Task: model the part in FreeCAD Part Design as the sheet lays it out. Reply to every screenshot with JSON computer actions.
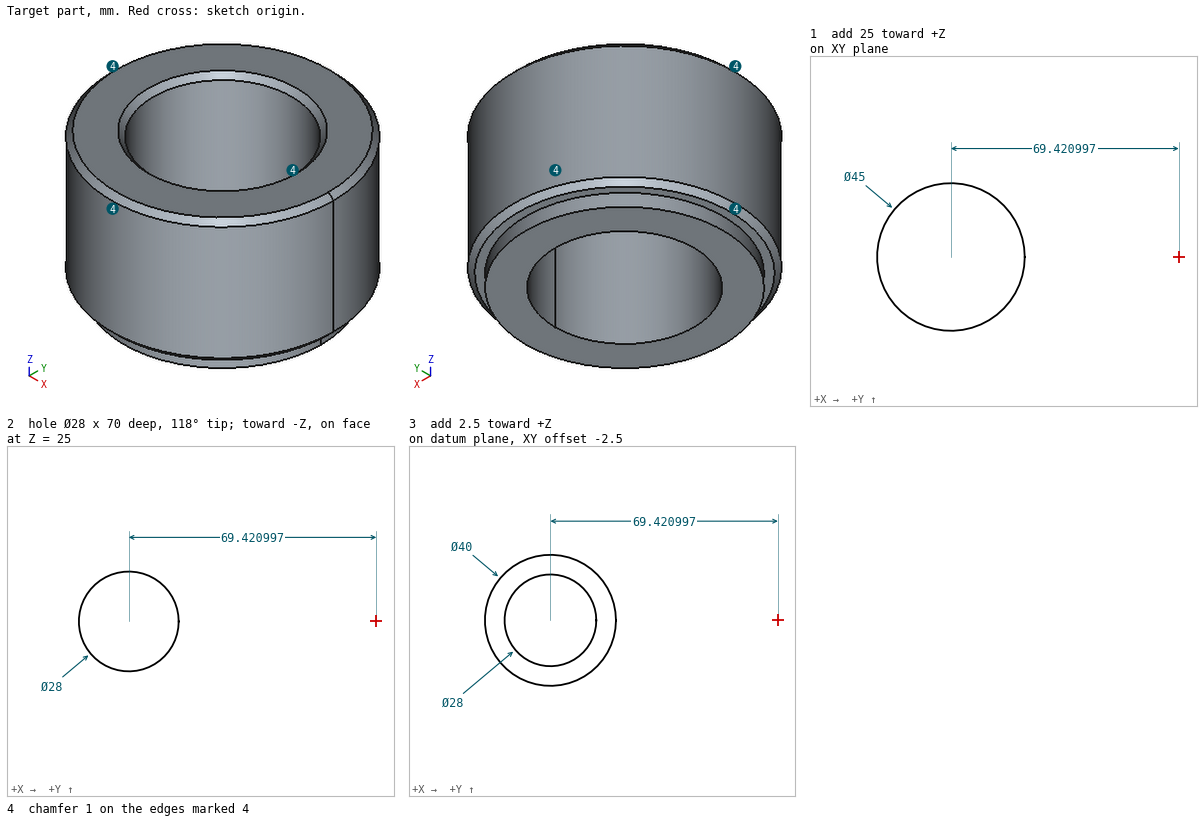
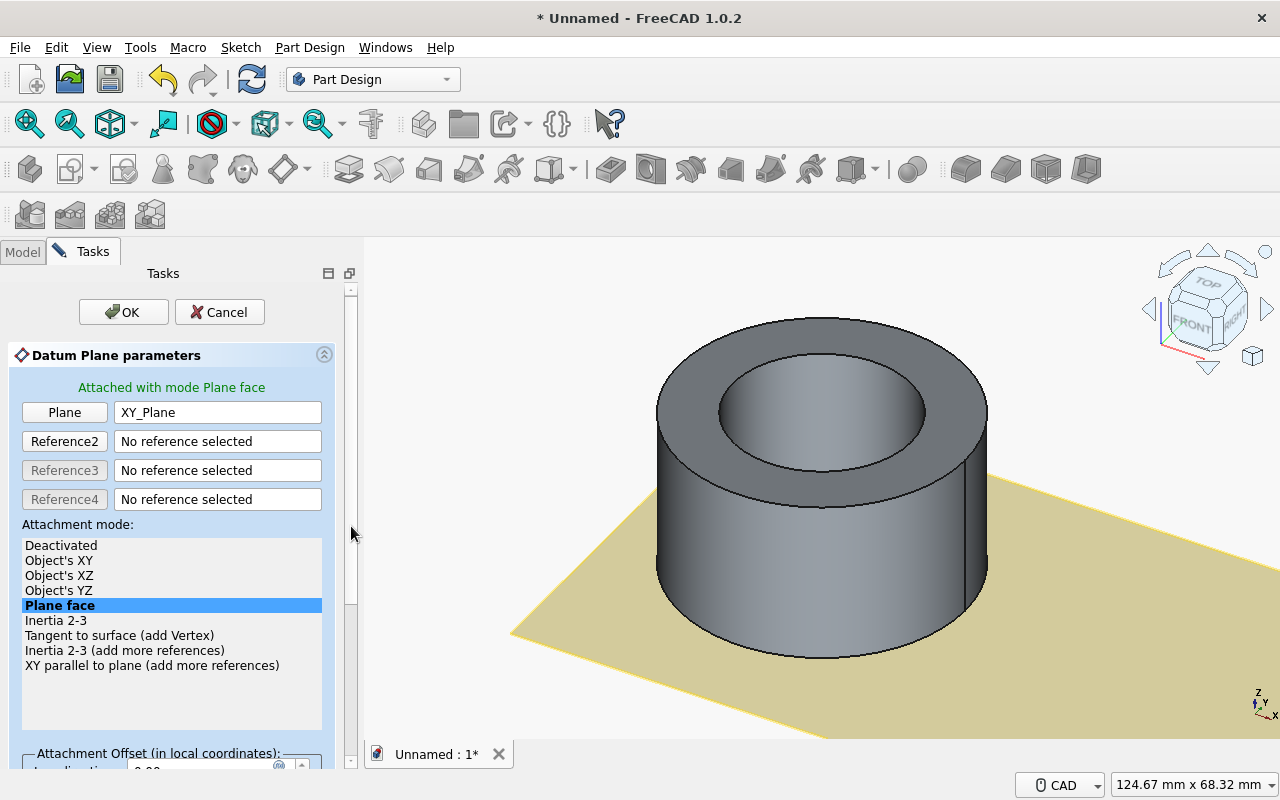
{"action": "left_click", "coordinate": [124, 312]}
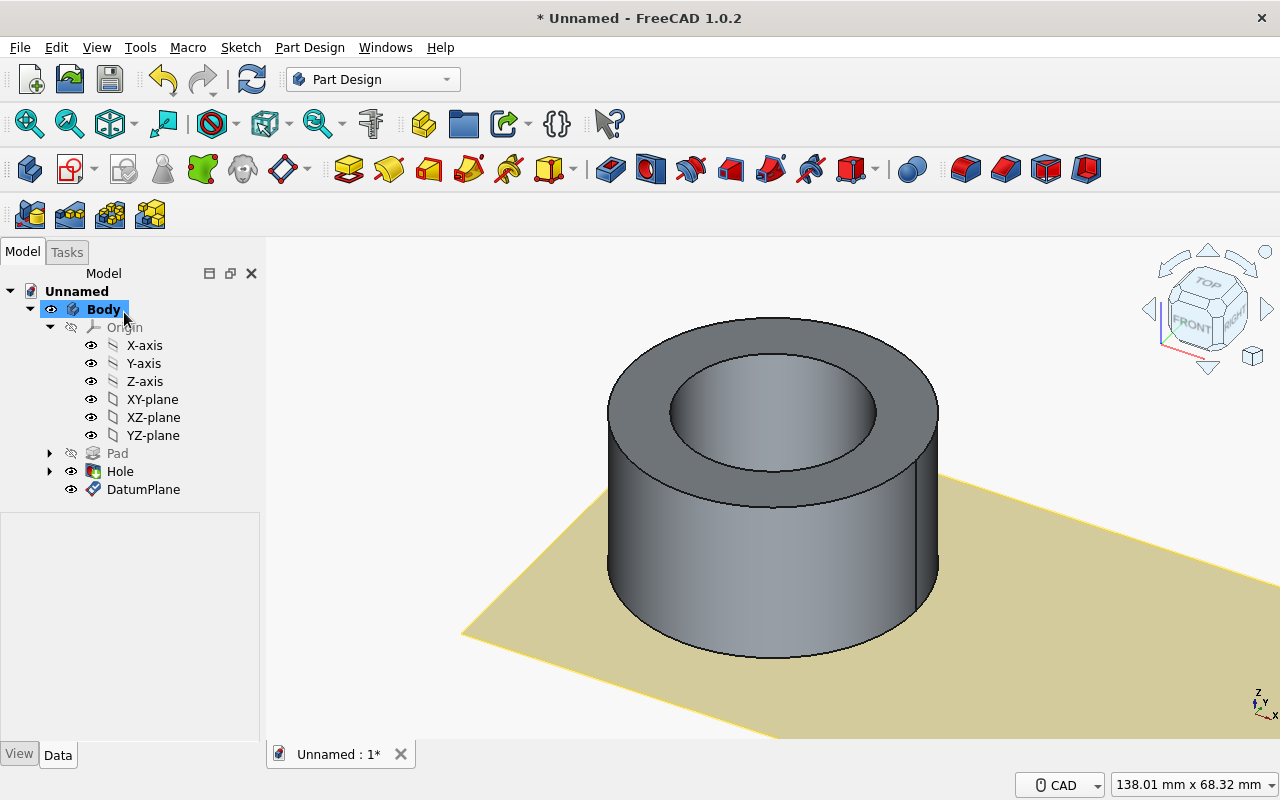
{"action": "left_click", "coordinate": [116, 489]}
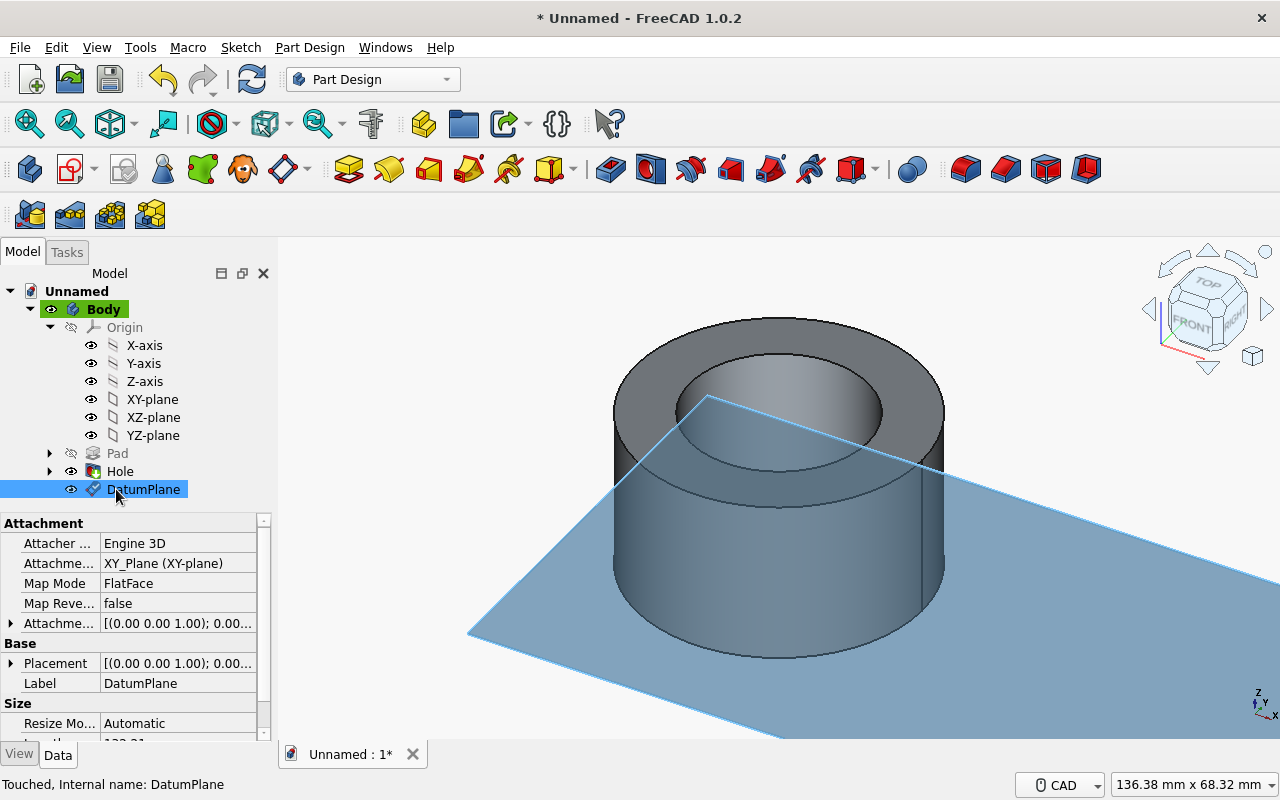
{"action": "left_click", "coordinate": [70, 170]}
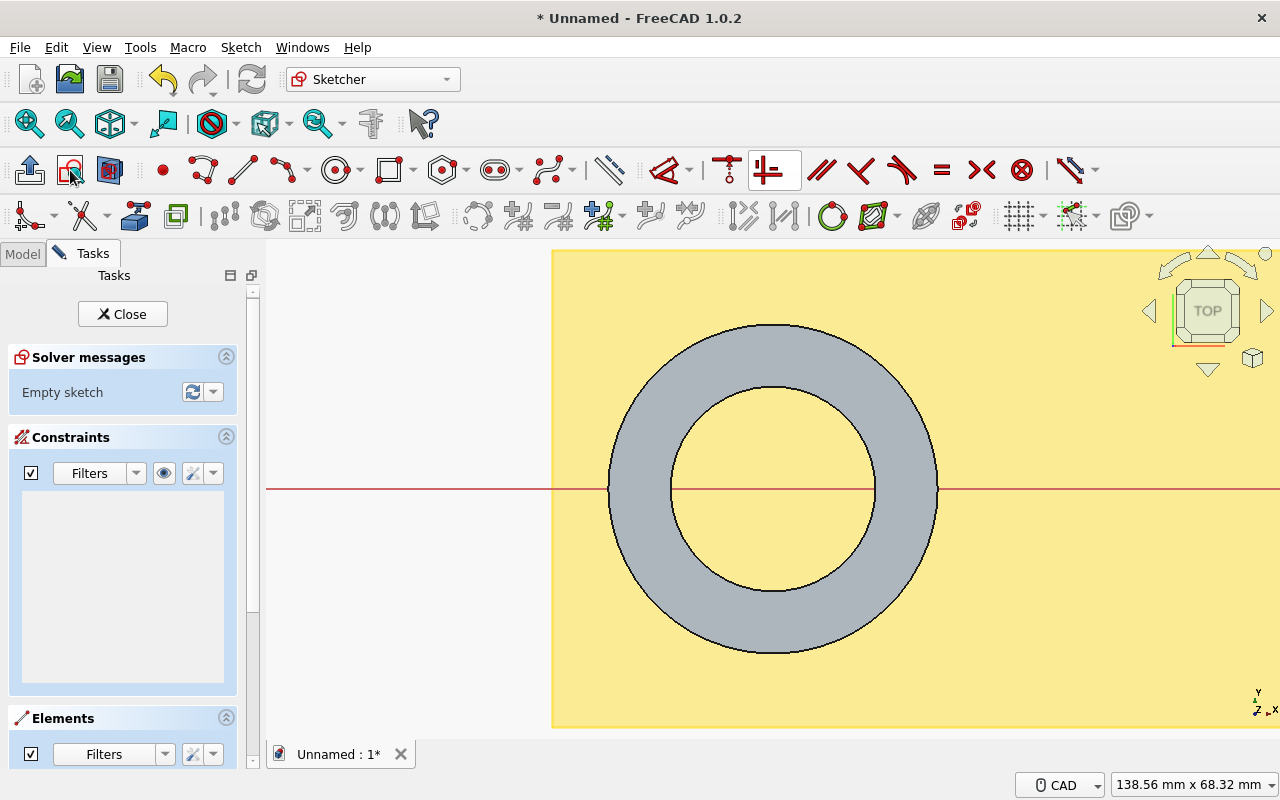
{"action": "left_click", "coordinate": [110, 170]}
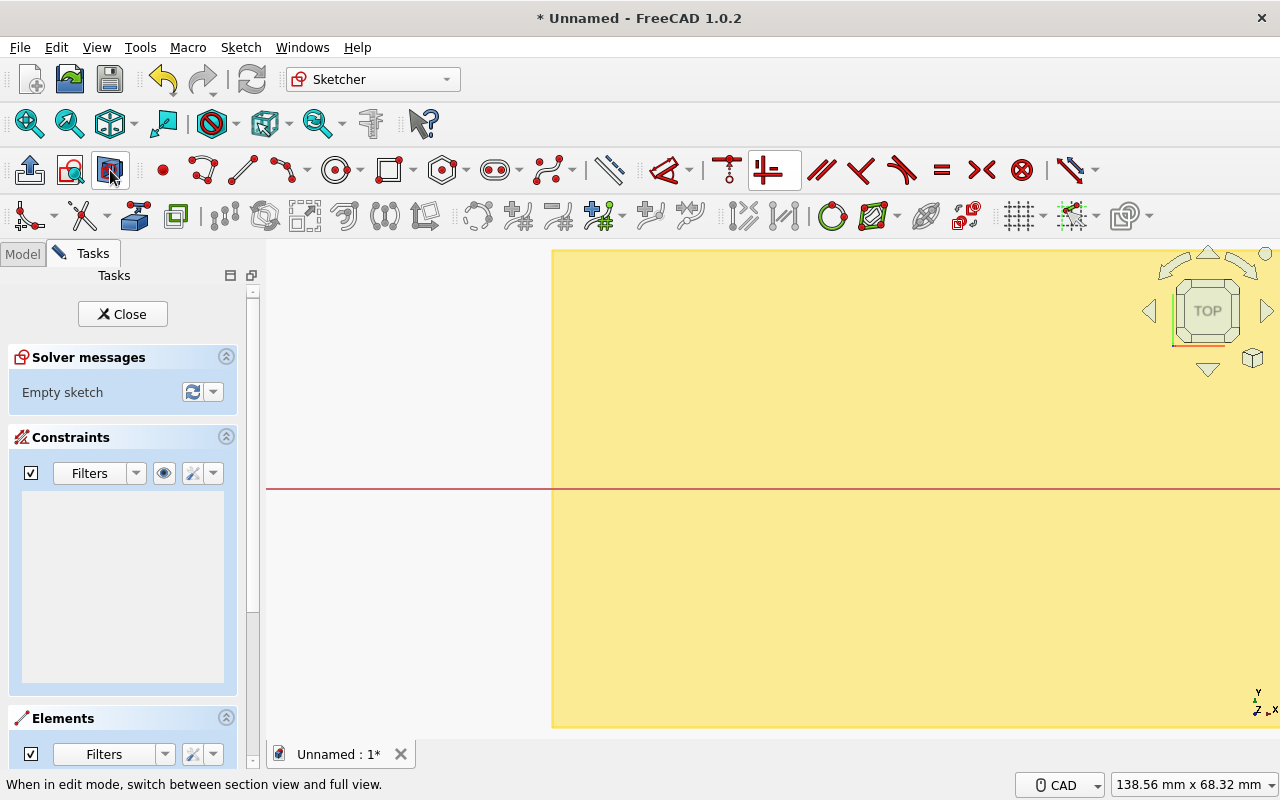
{"action": "scroll", "coordinate": [294, 489], "scroll_direction": "down", "scroll_amount": 2}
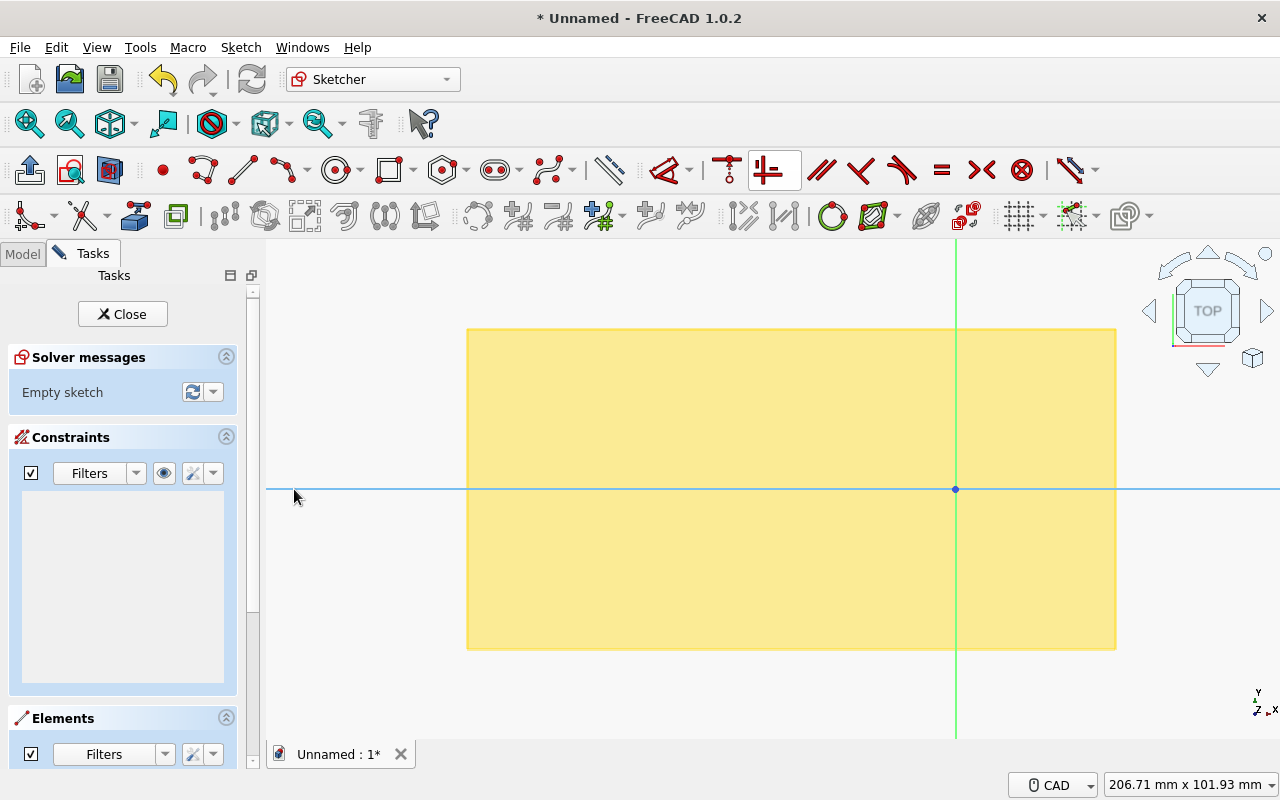
{"action": "key", "text": "g c"}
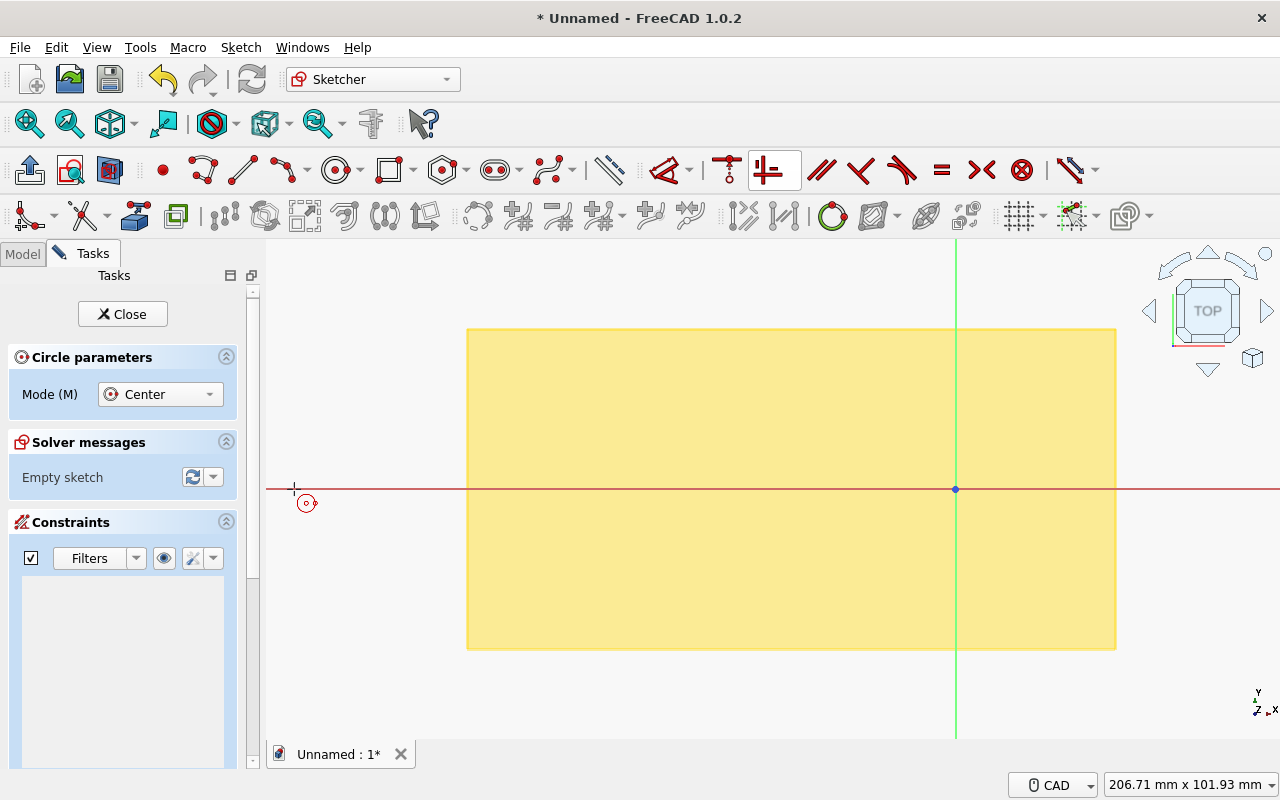
{"action": "left_click", "coordinate": [615, 489]}
{"action": "mouse_move", "coordinate": [684, 420]}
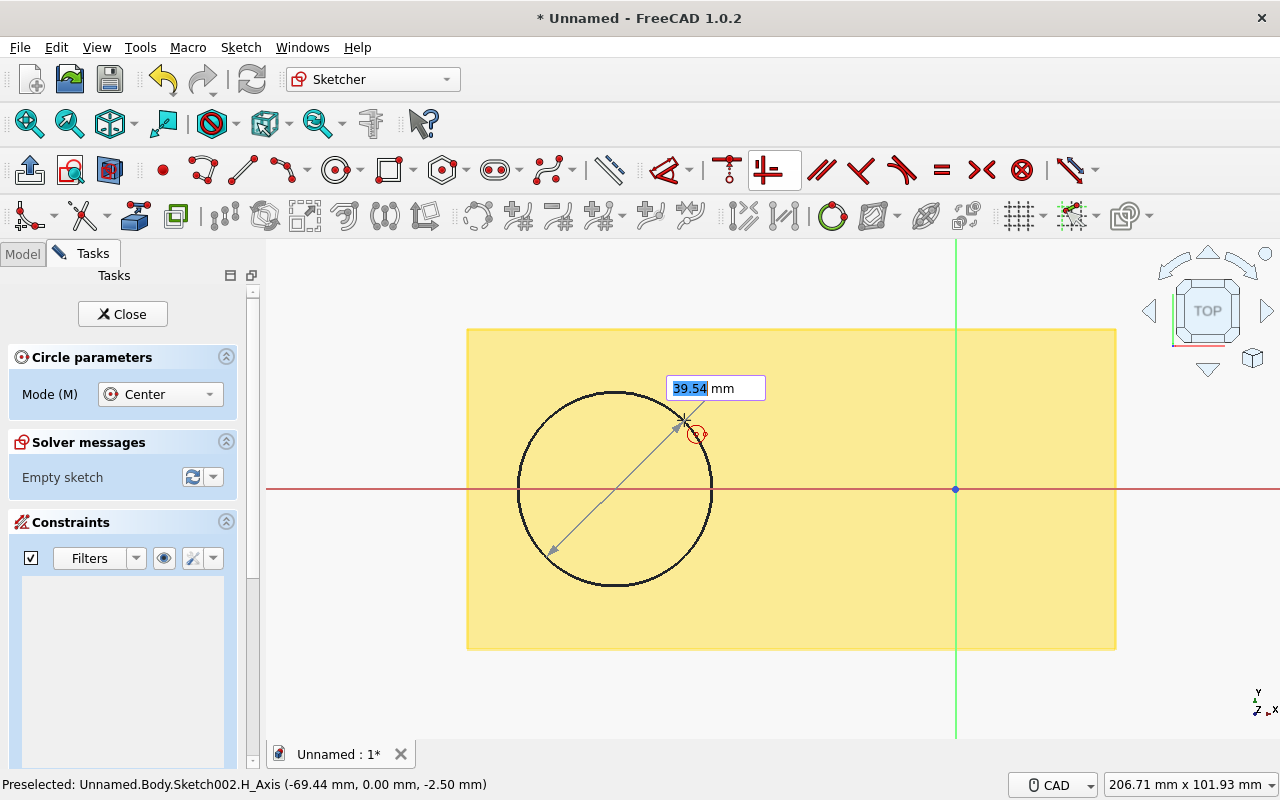
{"action": "type", "text": "40"}
{"action": "key", "text": "Return"}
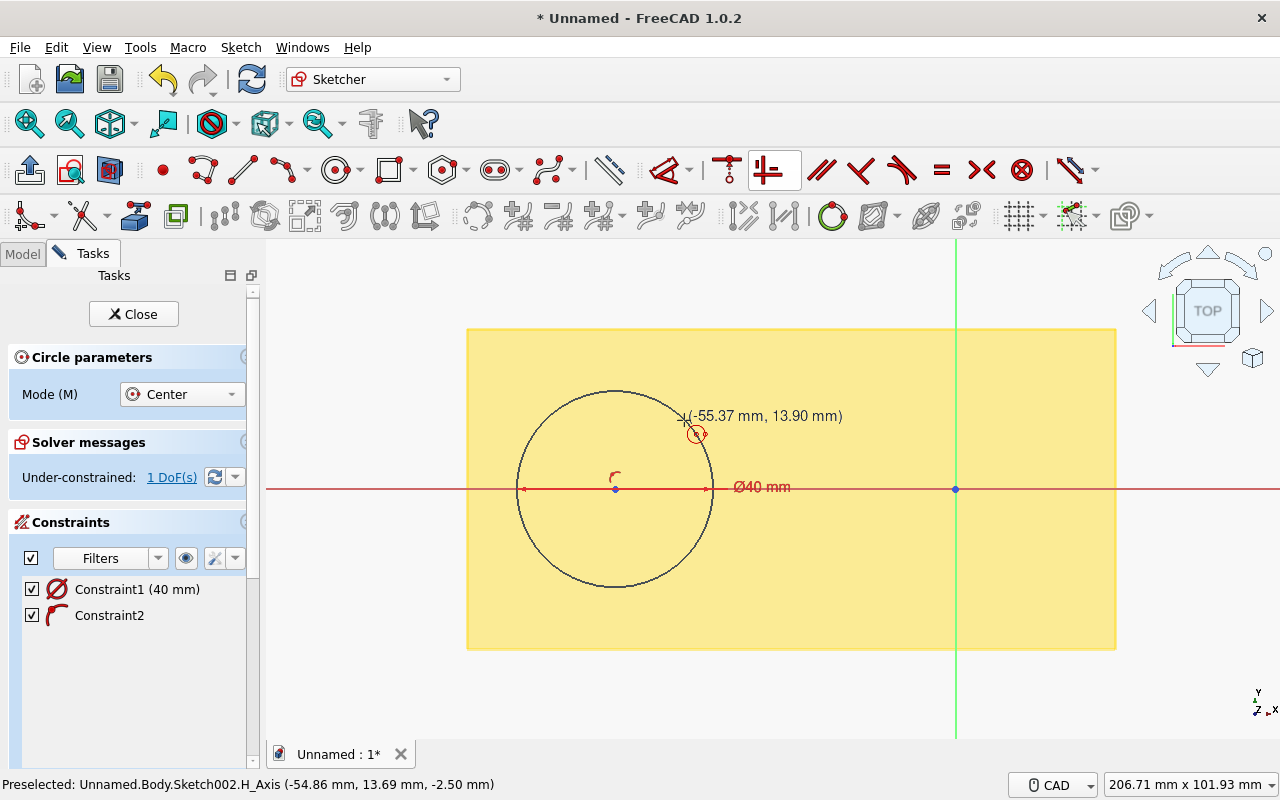
{"action": "left_click", "coordinate": [615, 489]}
{"action": "mouse_move", "coordinate": [664, 441]}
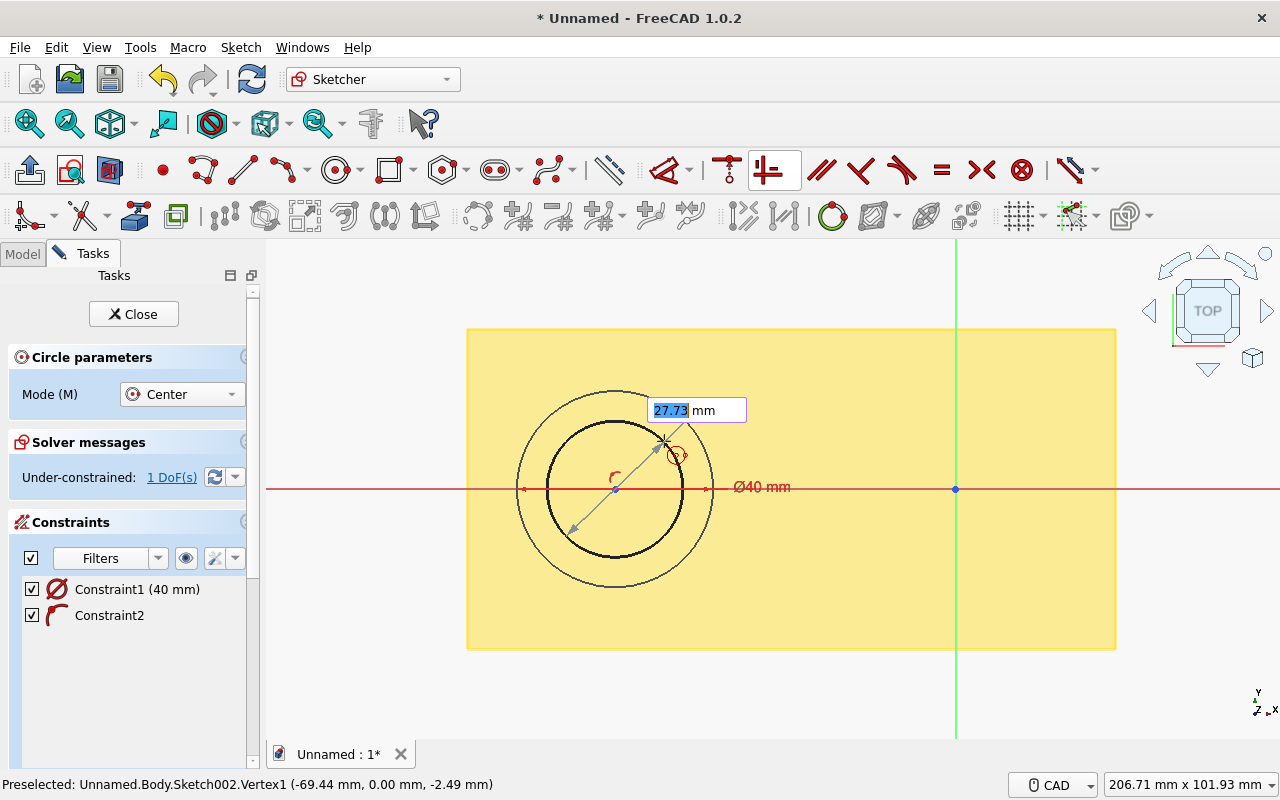
{"action": "type", "text": "28"}
{"action": "key", "text": "Return"}
{"action": "key", "text": "Escape"}